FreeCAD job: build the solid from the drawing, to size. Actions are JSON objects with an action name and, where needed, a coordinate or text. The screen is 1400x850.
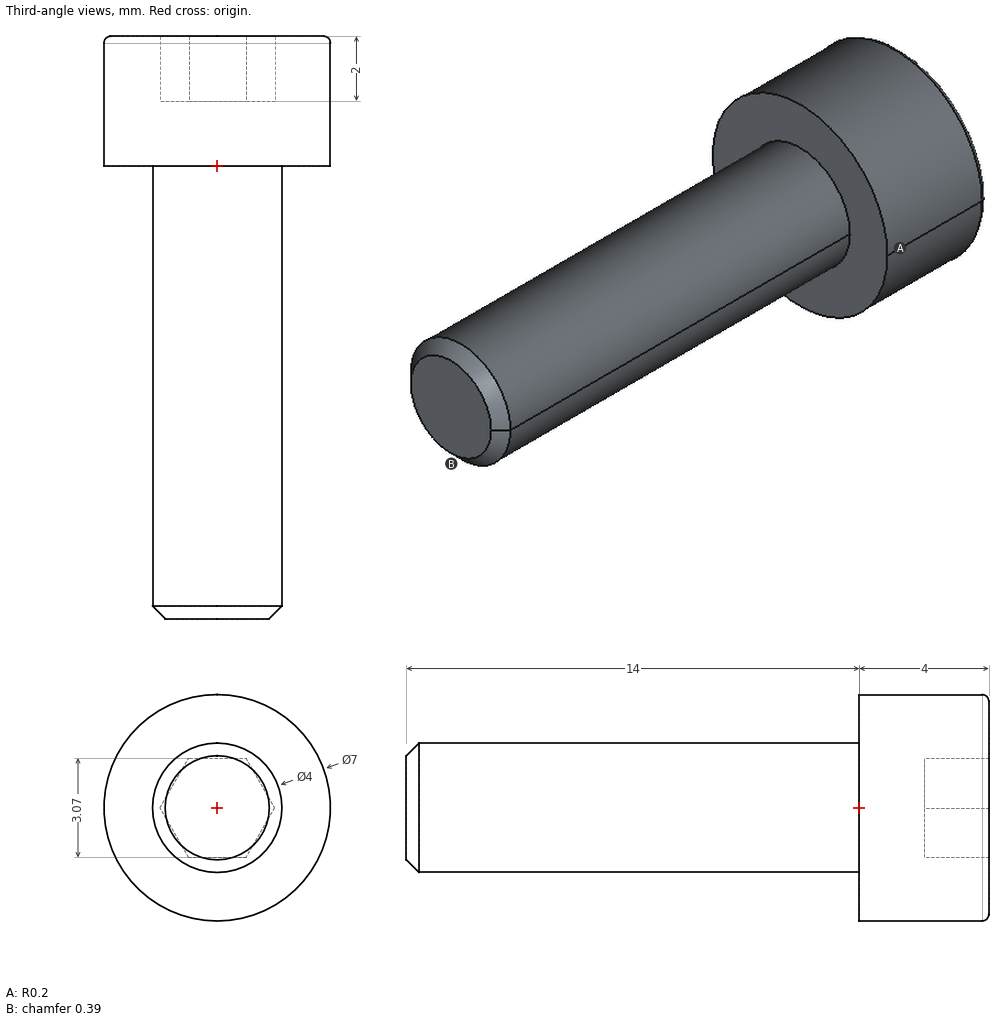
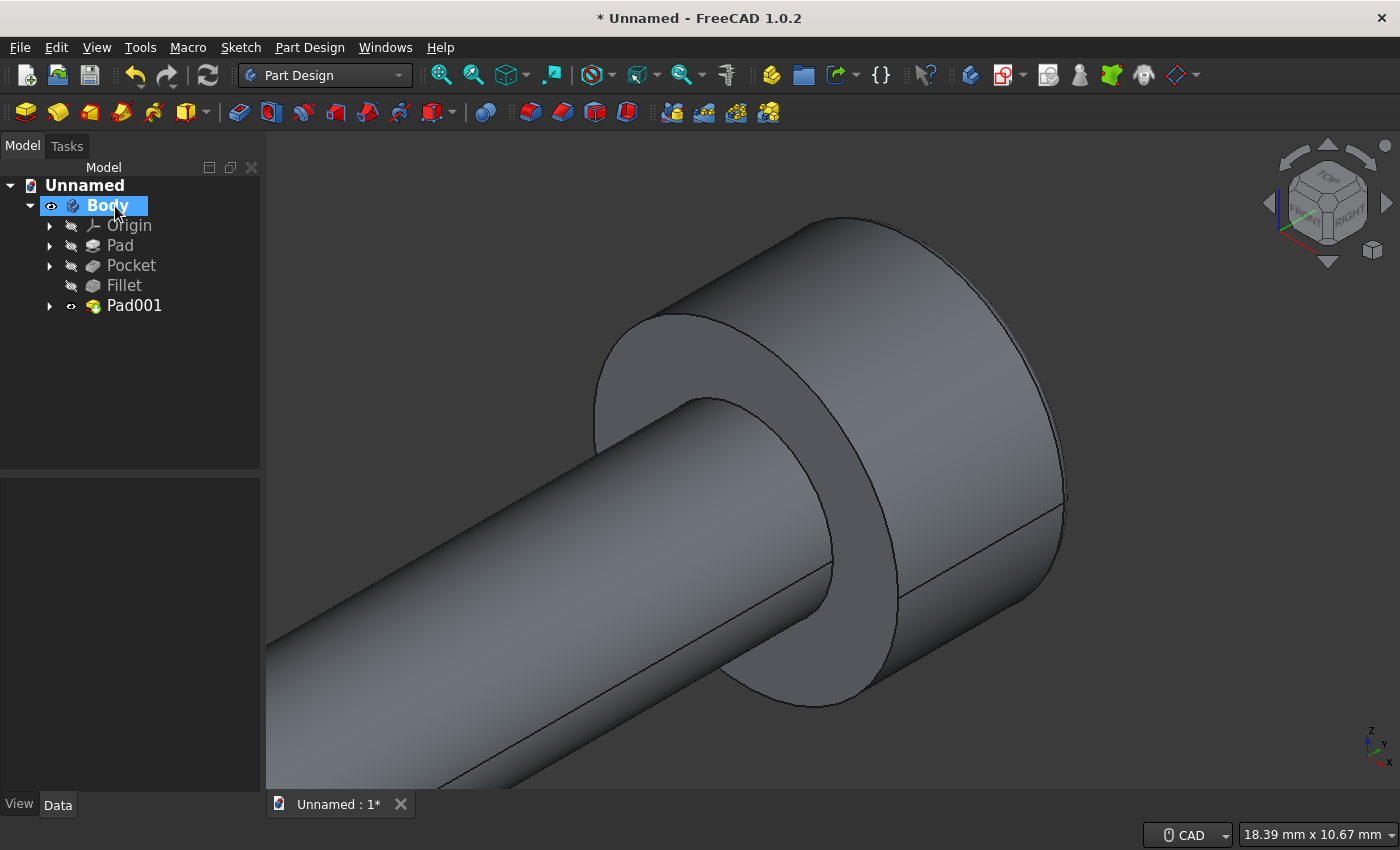
{"action": "left_click", "coordinate": [442, 76]}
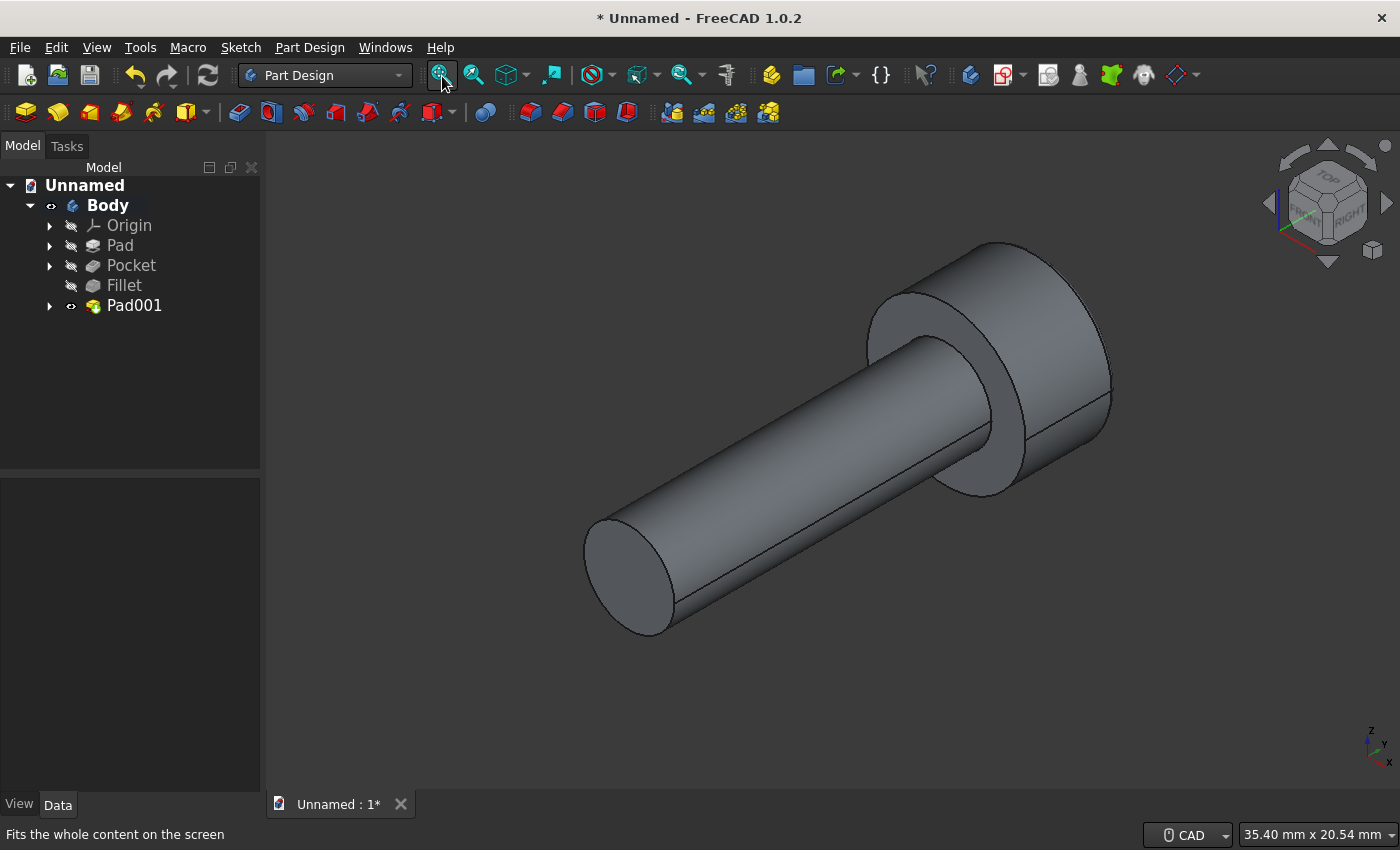
{"action": "left_click", "coordinate": [615, 519]}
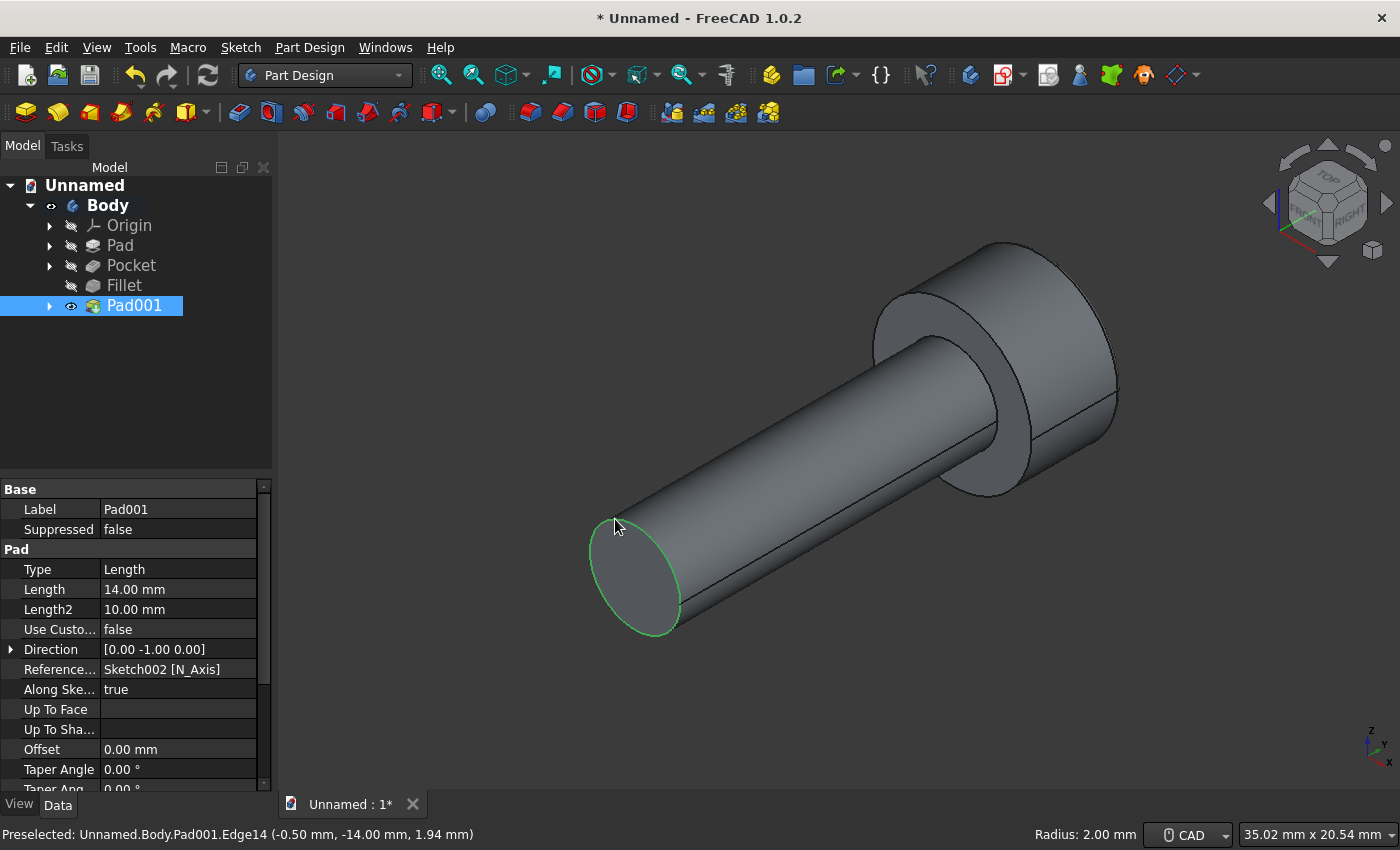
{"action": "left_click", "coordinate": [564, 112]}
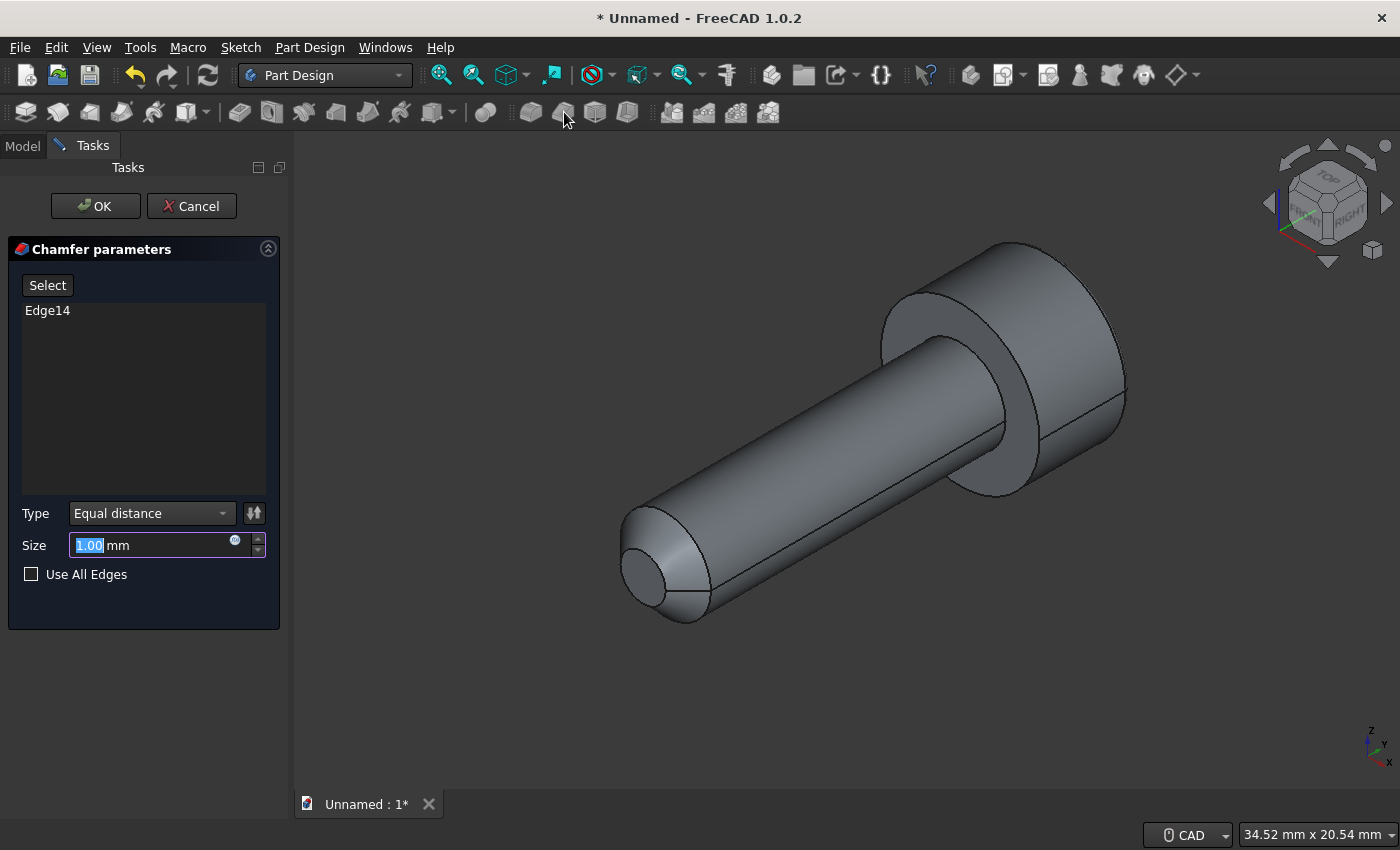
{"action": "type", "text": "0.39"}
{"action": "key", "text": "Tab"}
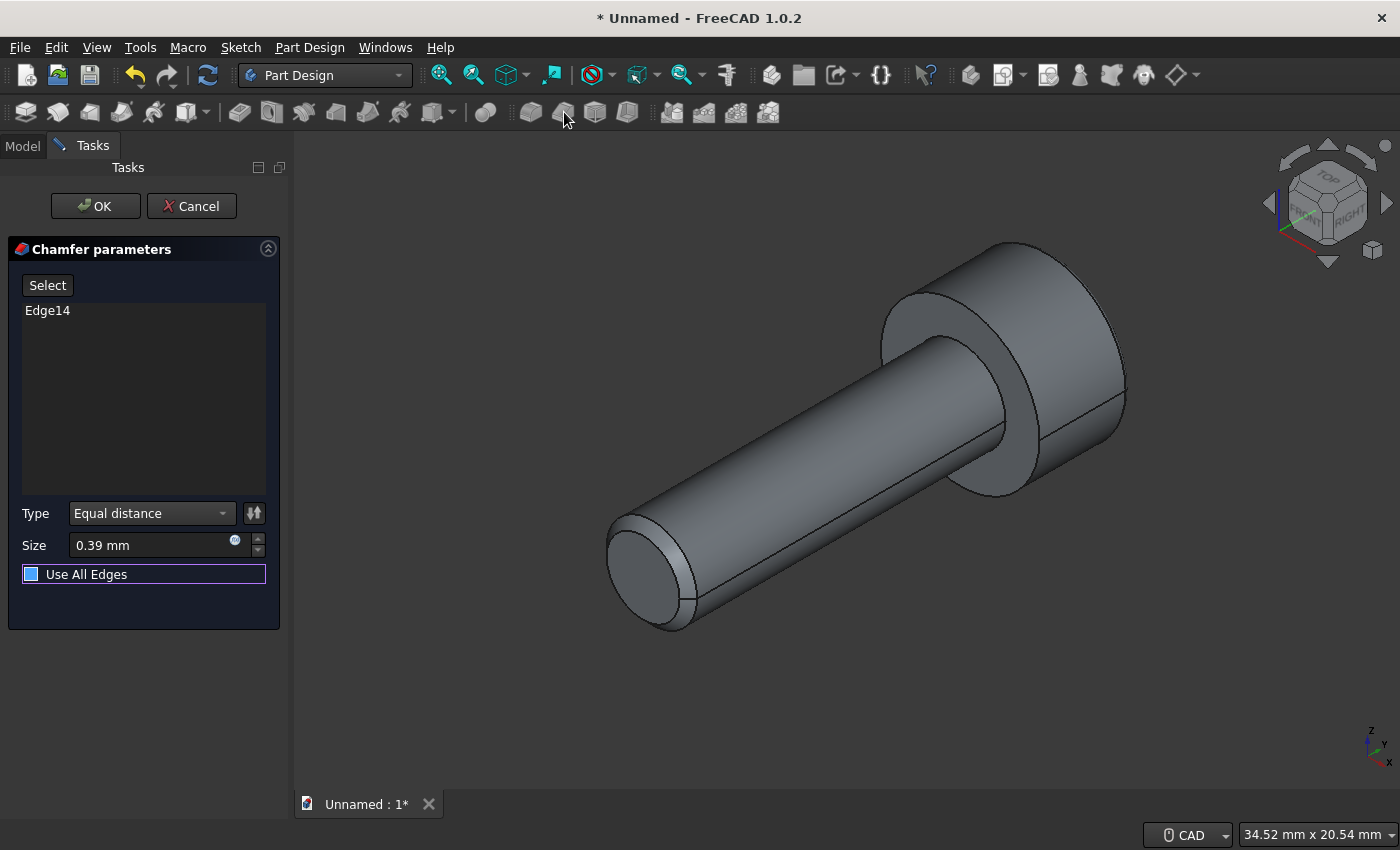
{"action": "left_click", "coordinate": [96, 206]}